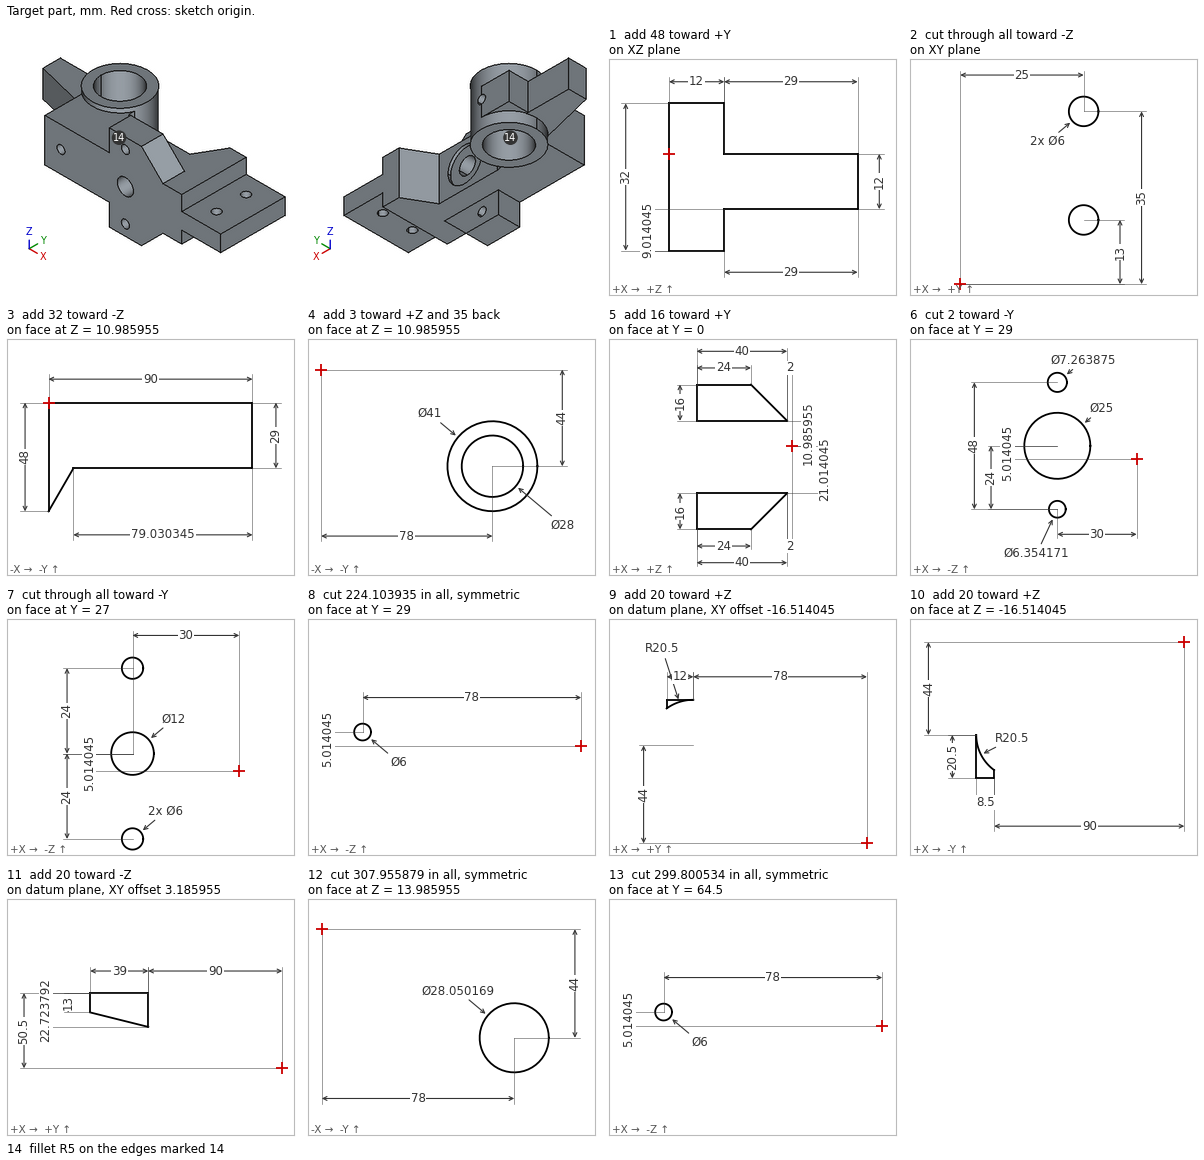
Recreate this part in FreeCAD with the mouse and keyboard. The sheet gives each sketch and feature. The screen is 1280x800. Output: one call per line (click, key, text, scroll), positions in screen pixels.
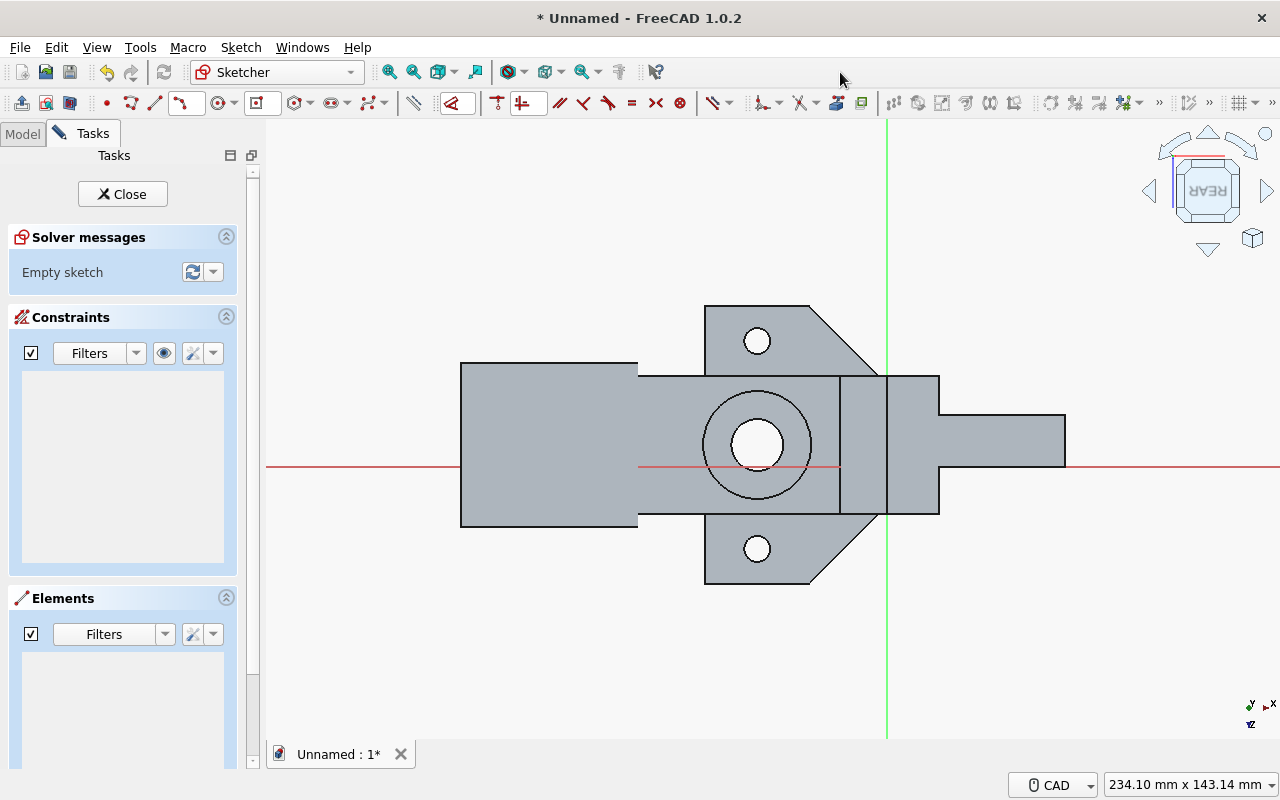
click(70, 104)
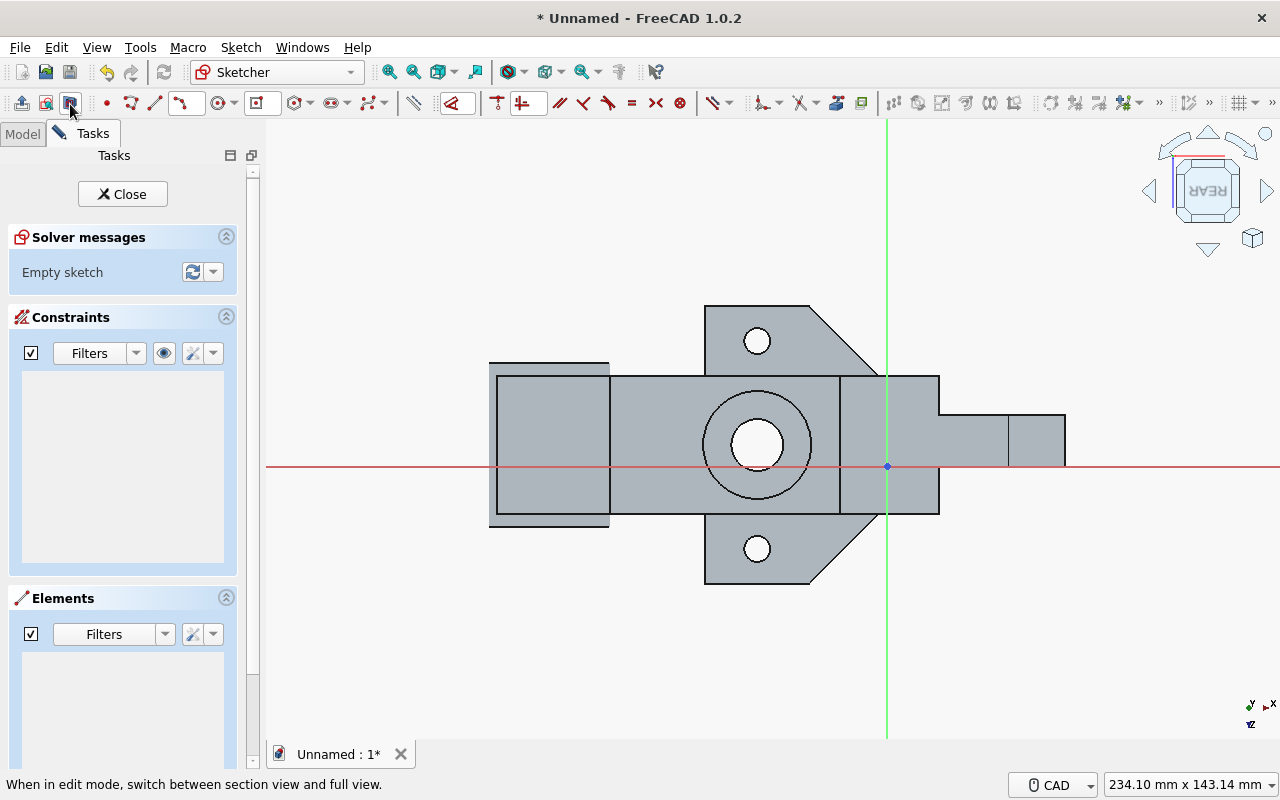
scroll(539, 446, up, 14)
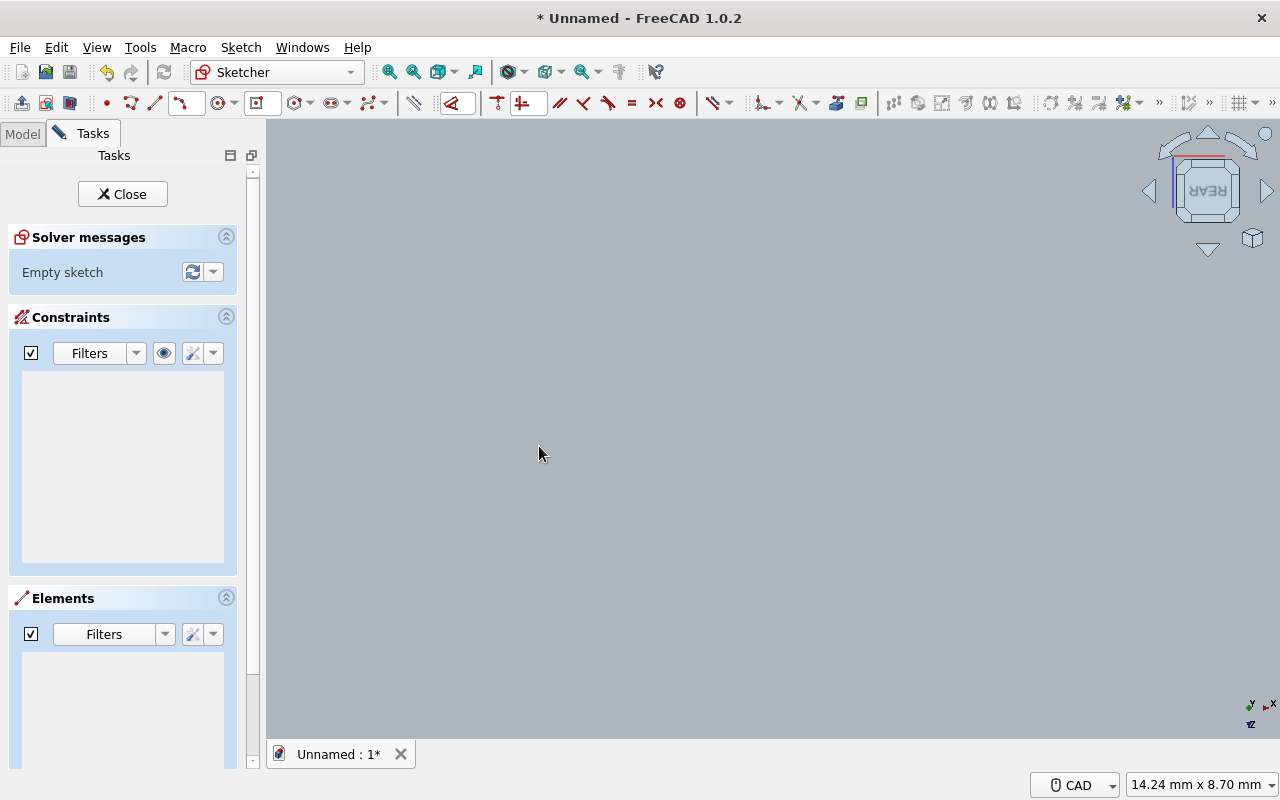
key(g)
key(c)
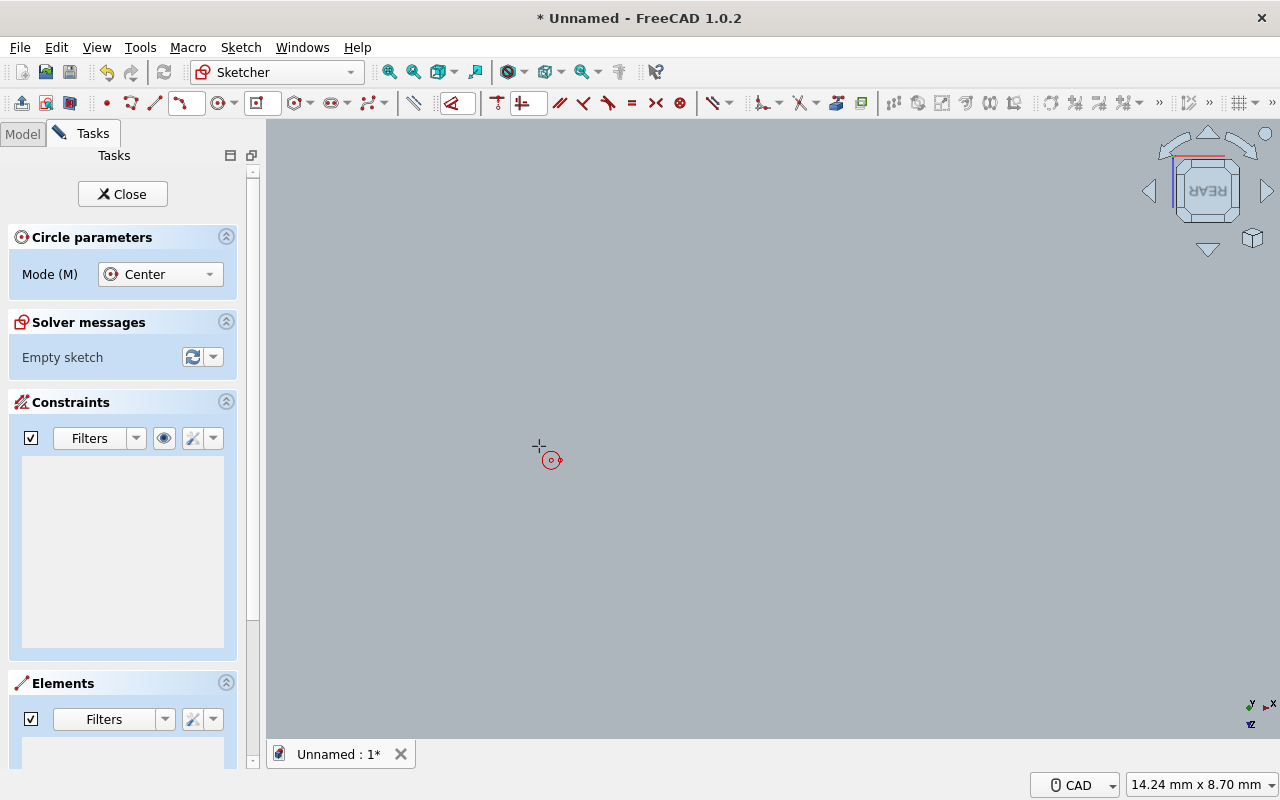
click(705, 421)
move(856, 270)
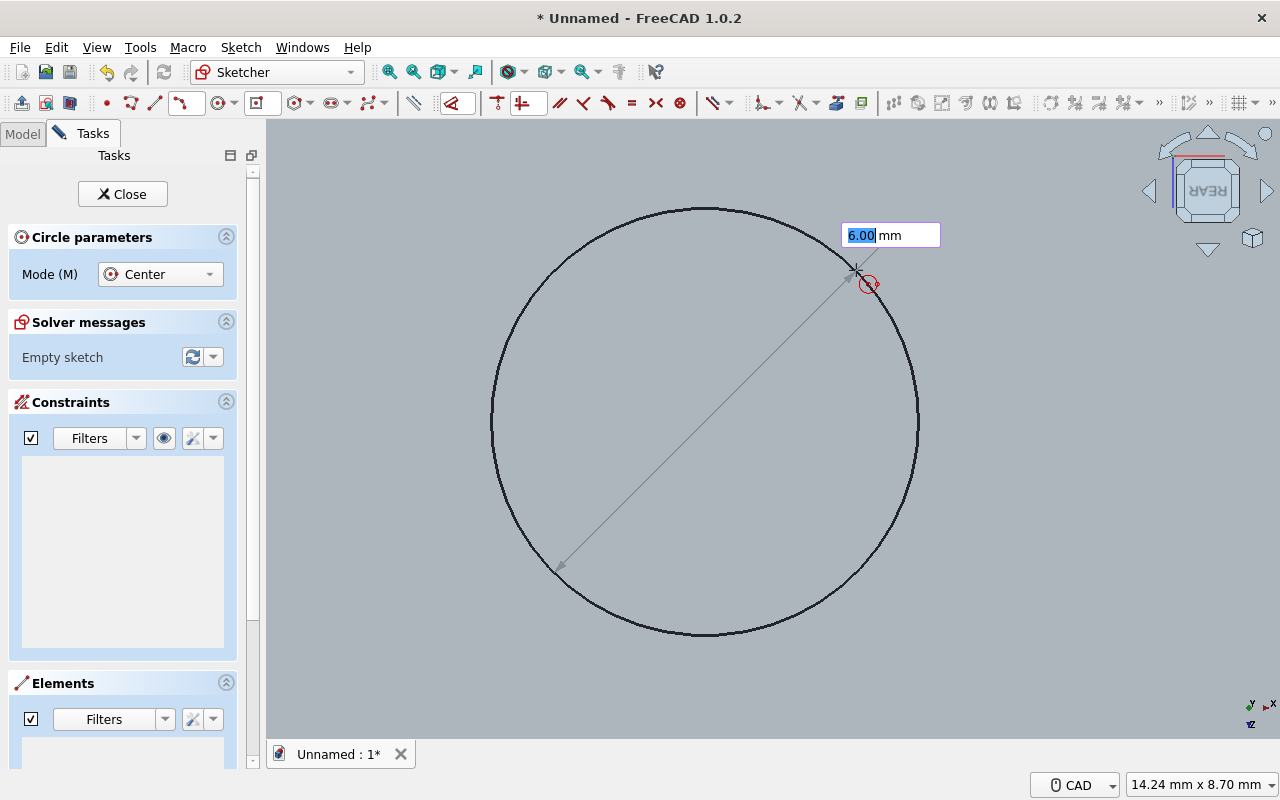
text(6)
key(Return)
key(Escape)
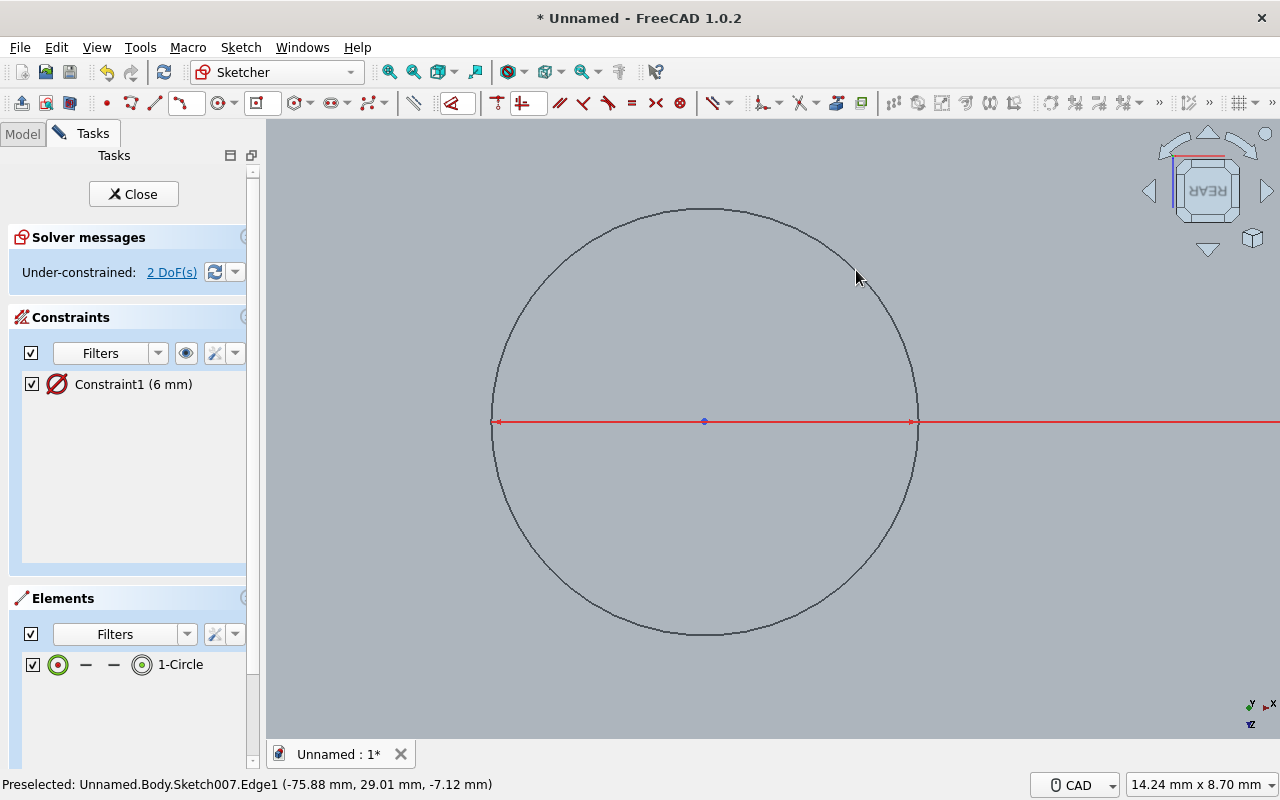
click(705, 422)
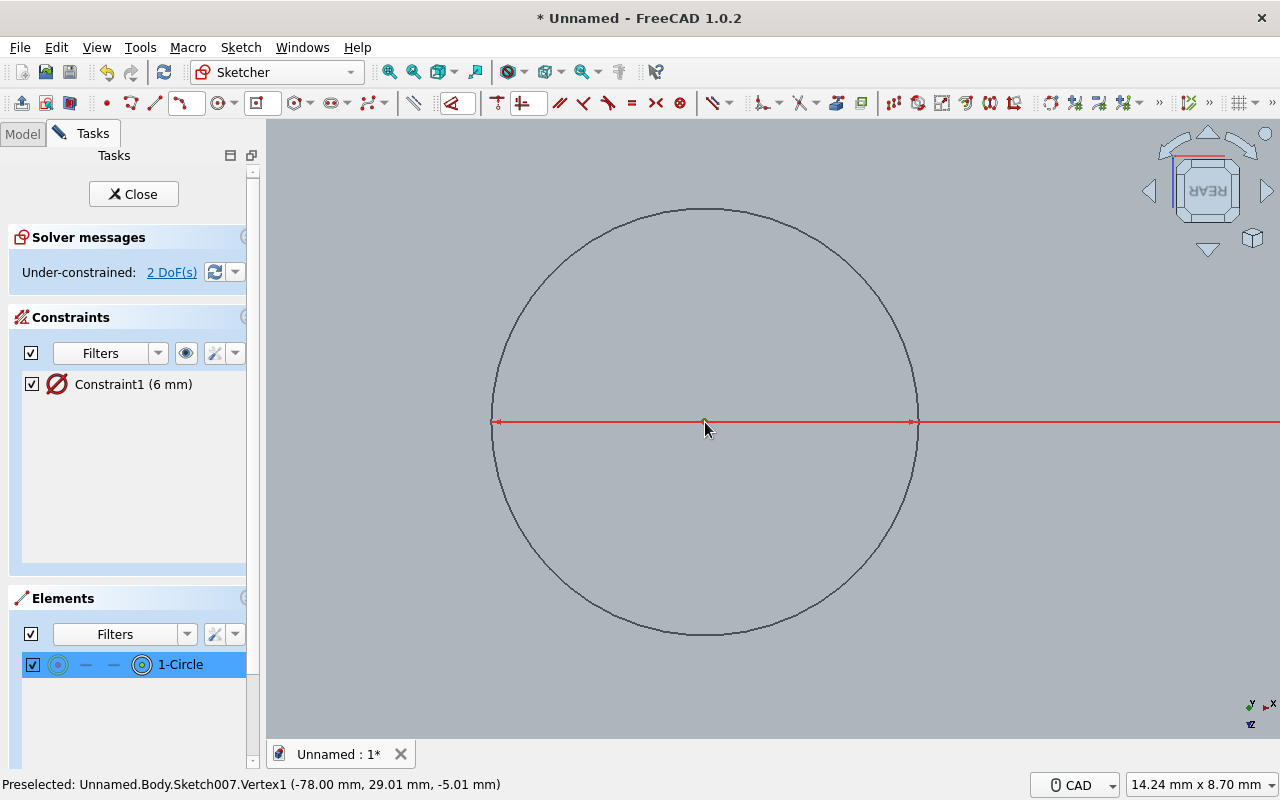
key(l)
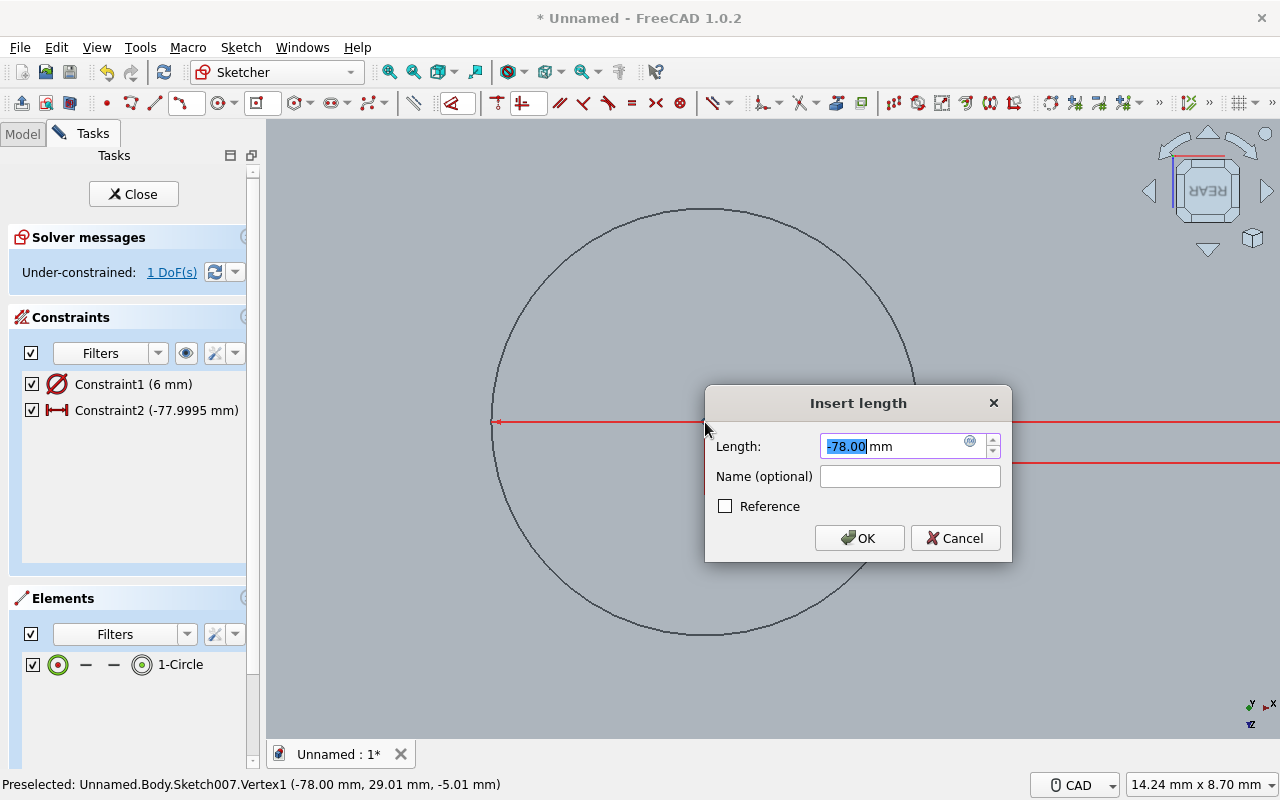
text(-78)
key(Return)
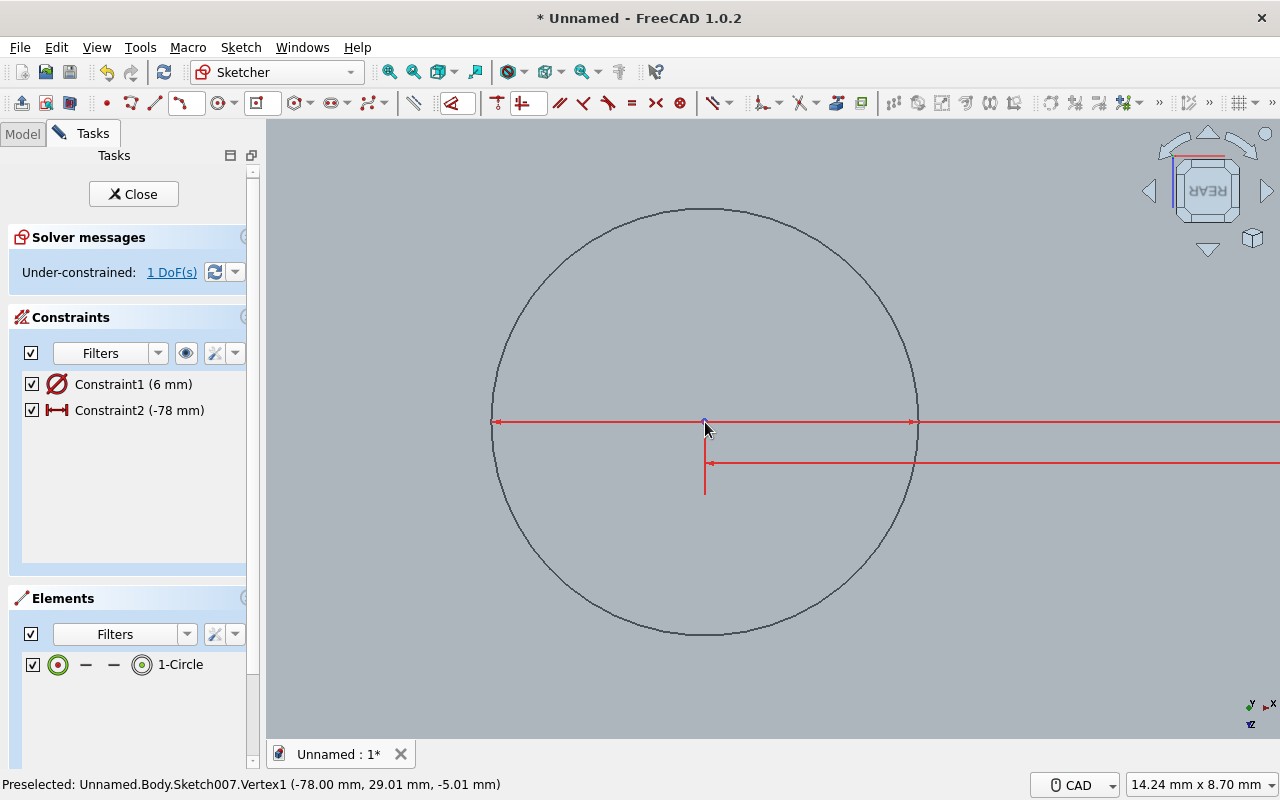
click(705, 422)